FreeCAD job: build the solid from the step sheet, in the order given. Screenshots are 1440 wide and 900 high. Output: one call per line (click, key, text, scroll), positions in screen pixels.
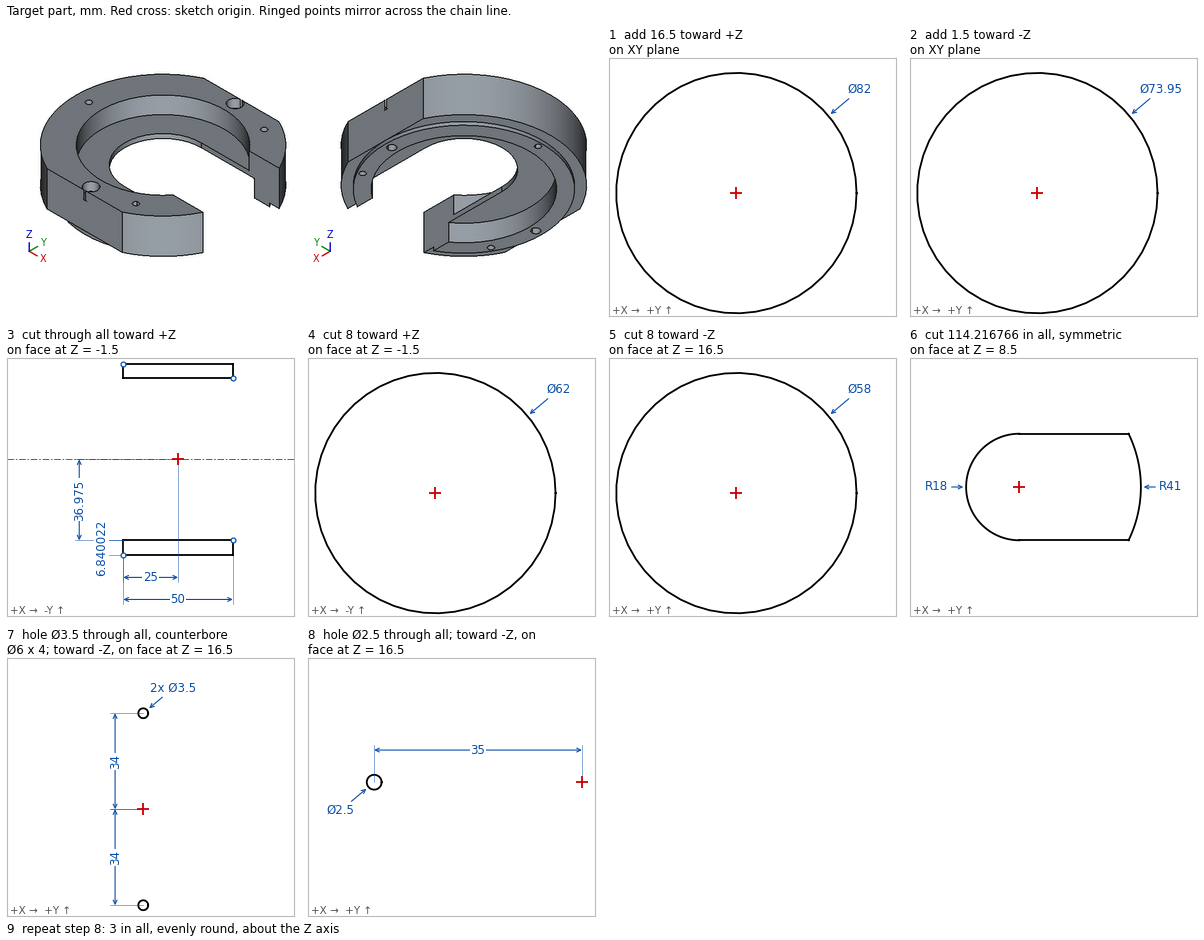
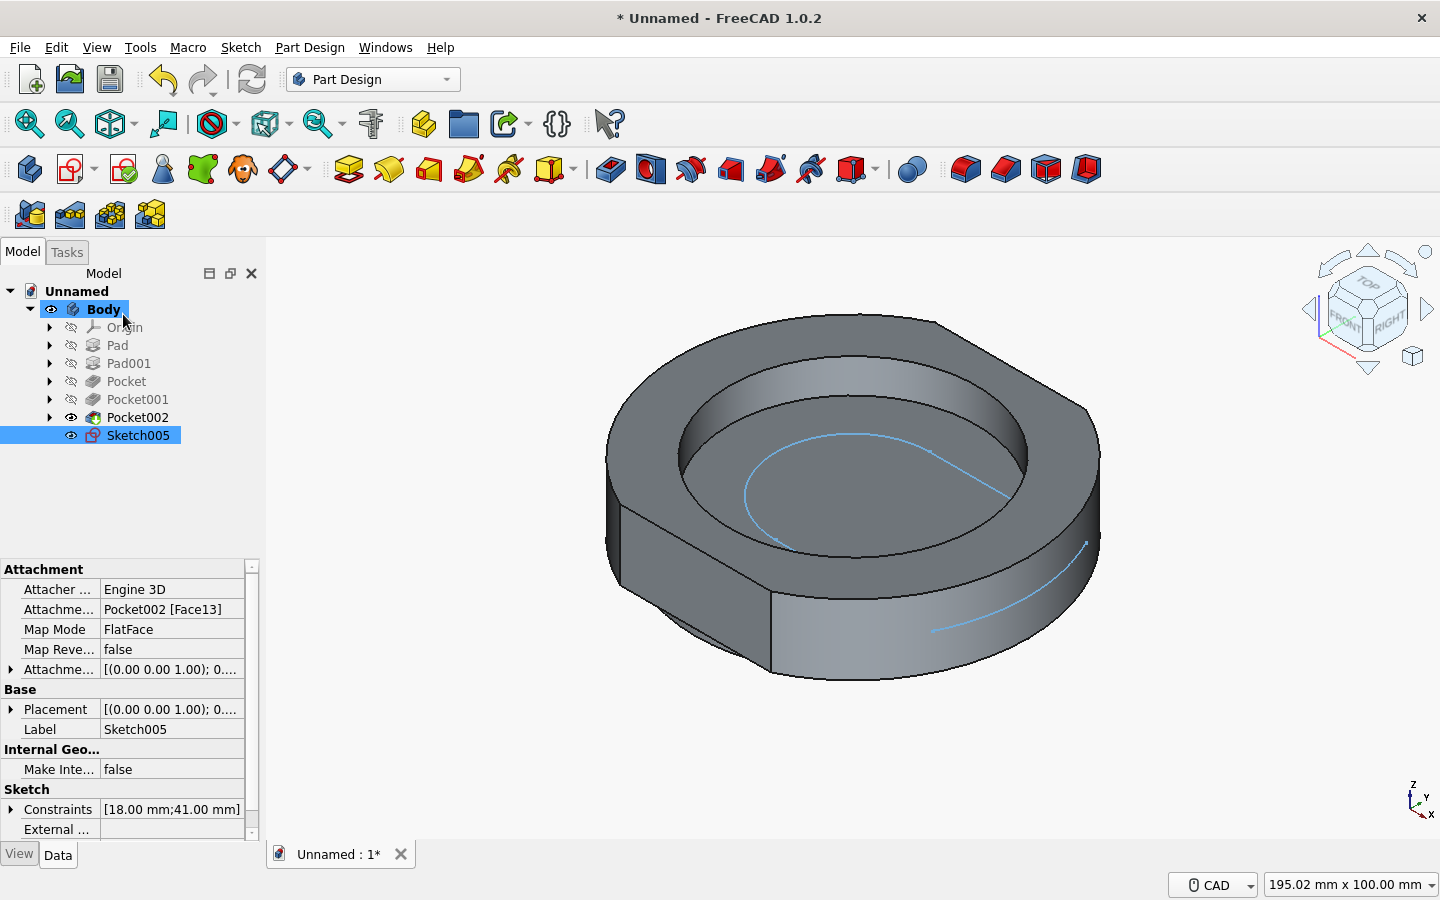
click(612, 170)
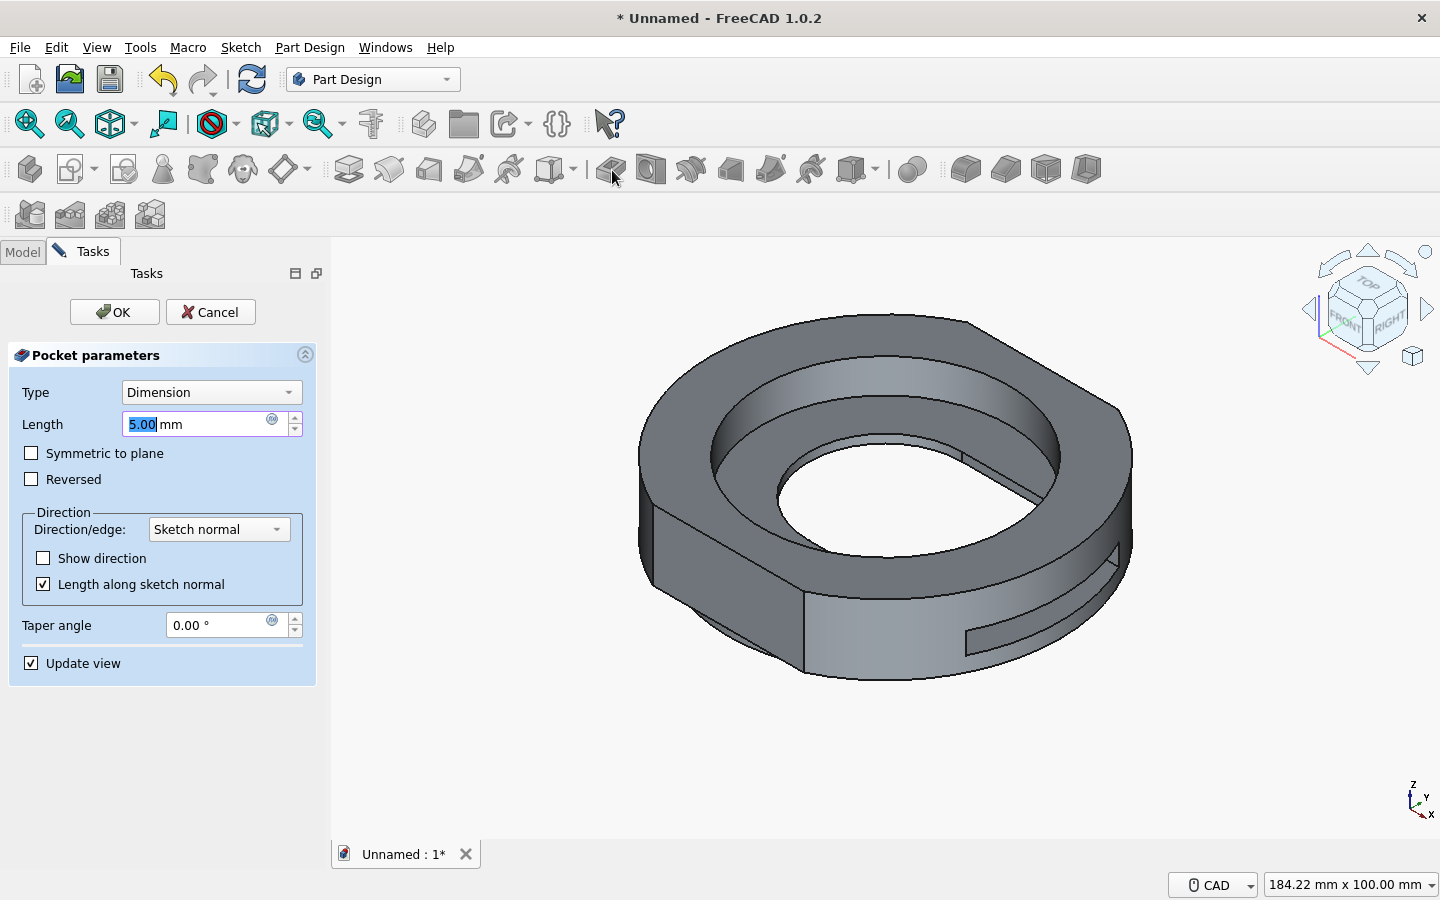
text(114.216766)
key(Tab)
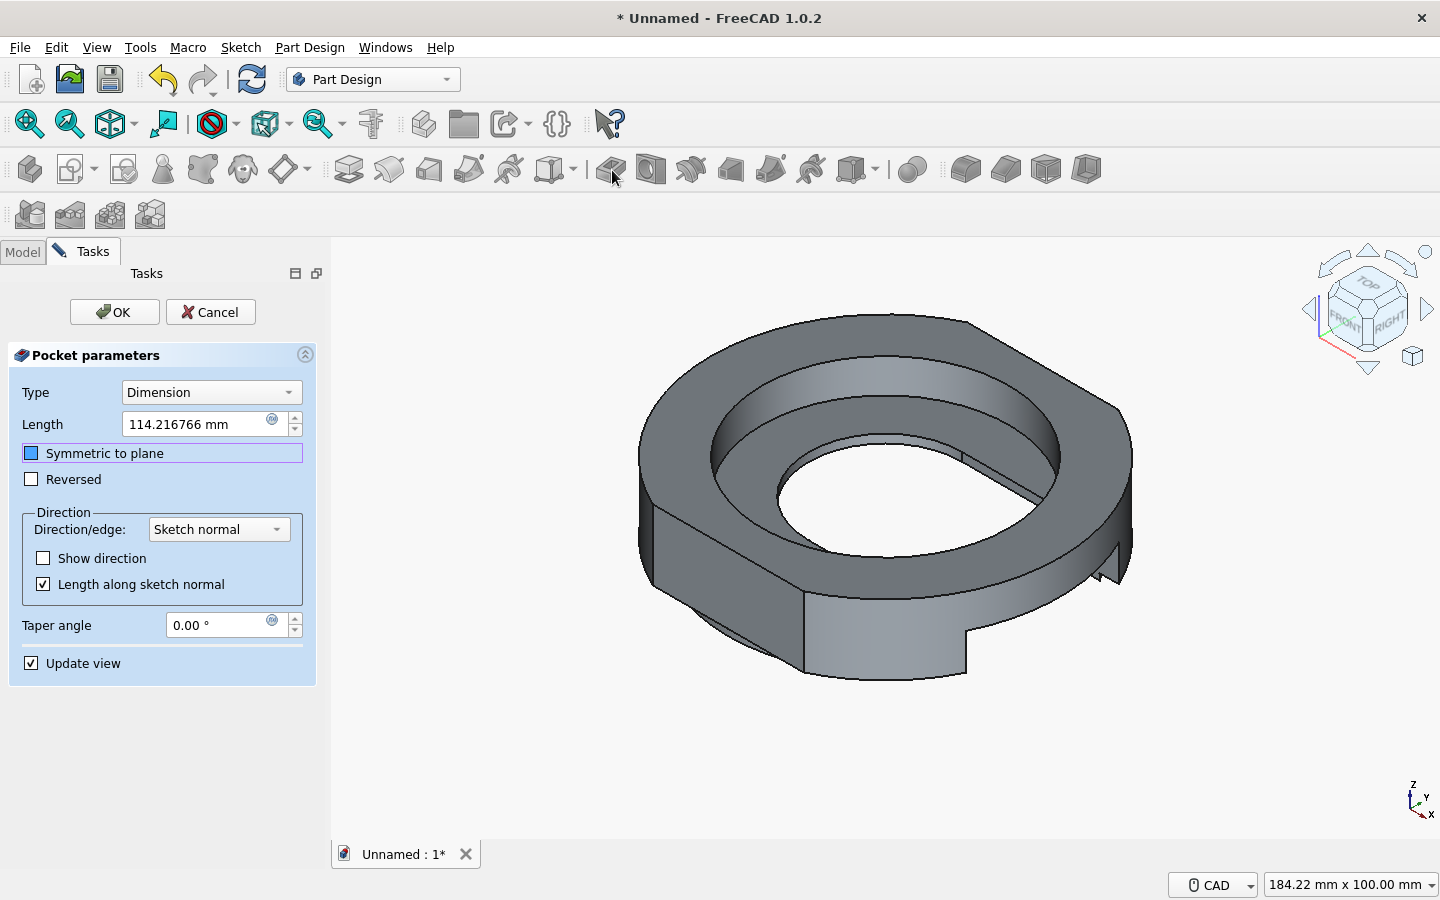
click(30, 453)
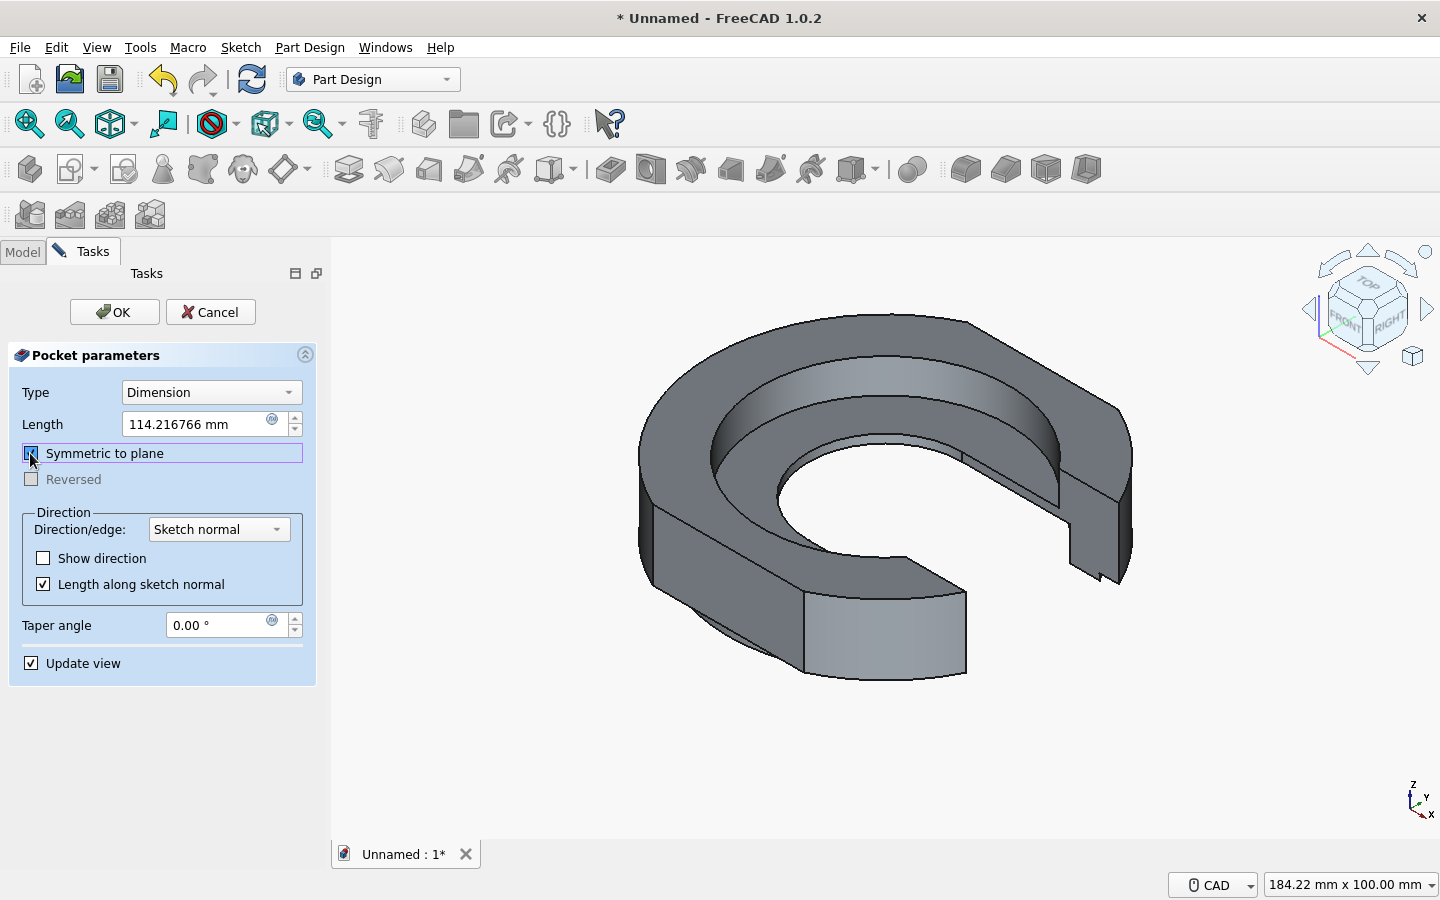
click(115, 312)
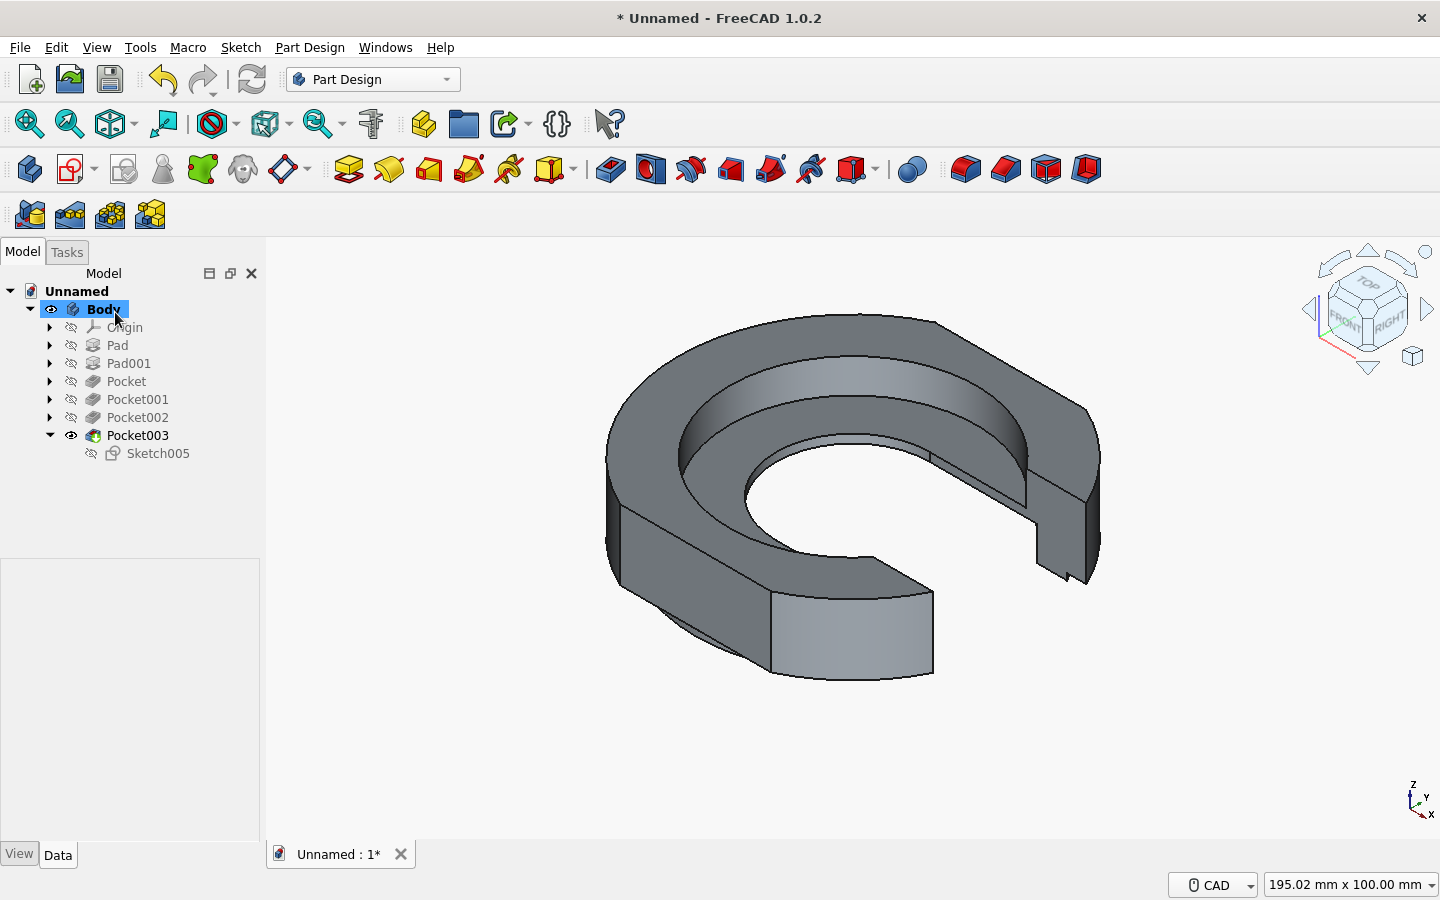
click(702, 369)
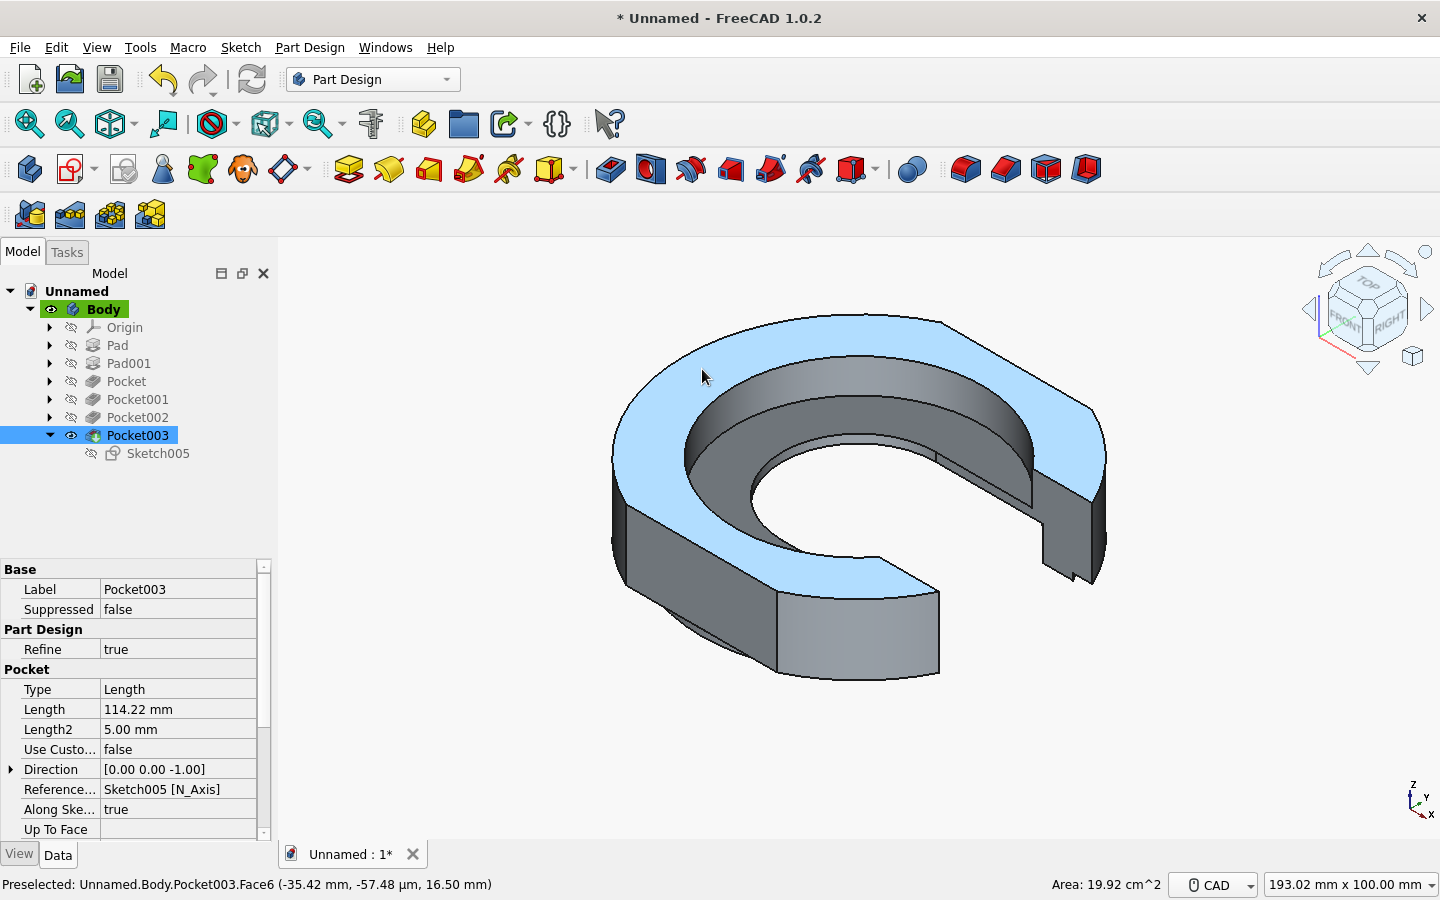
click(70, 170)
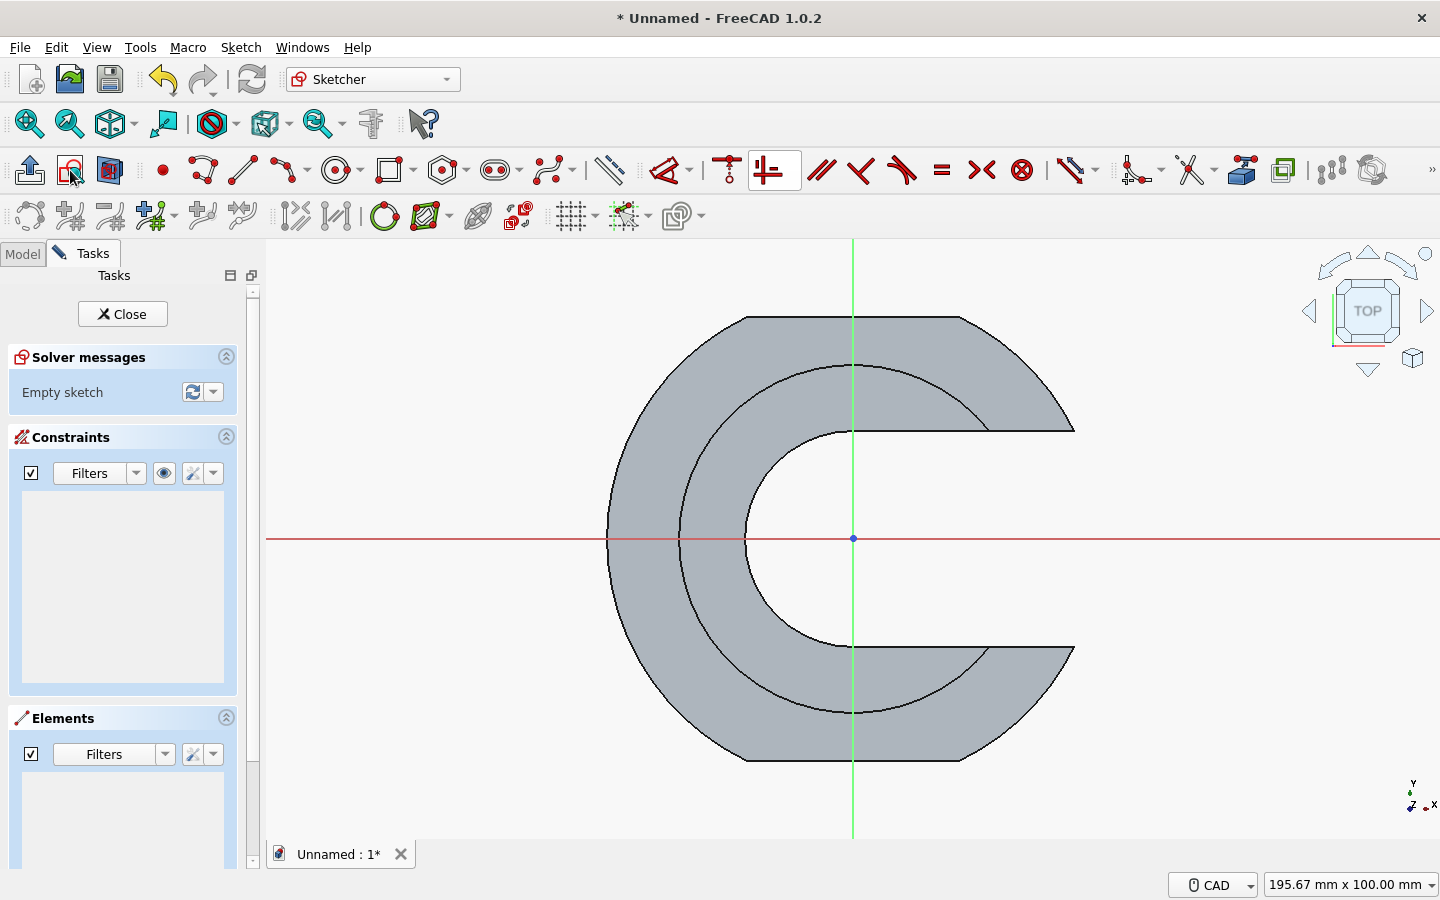
click(336, 170)